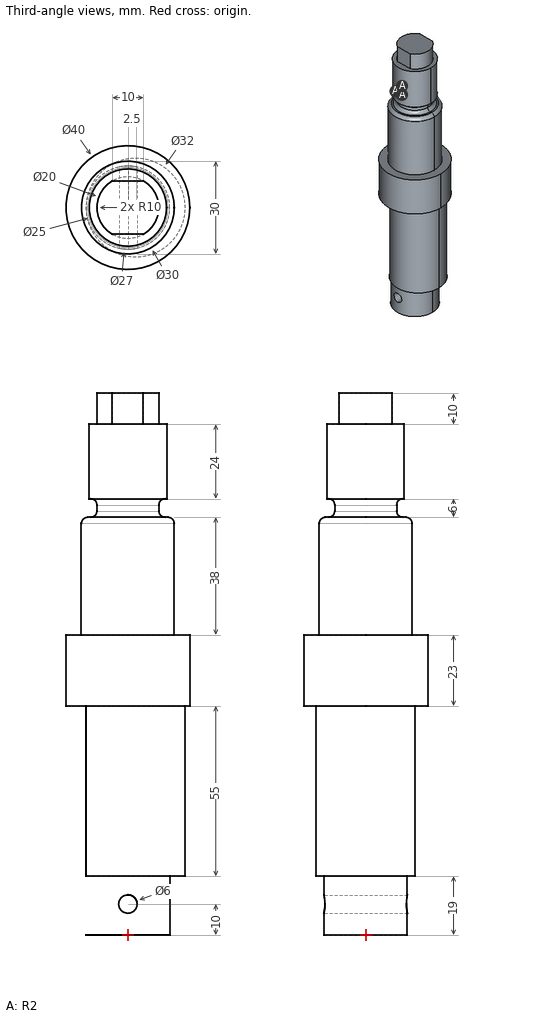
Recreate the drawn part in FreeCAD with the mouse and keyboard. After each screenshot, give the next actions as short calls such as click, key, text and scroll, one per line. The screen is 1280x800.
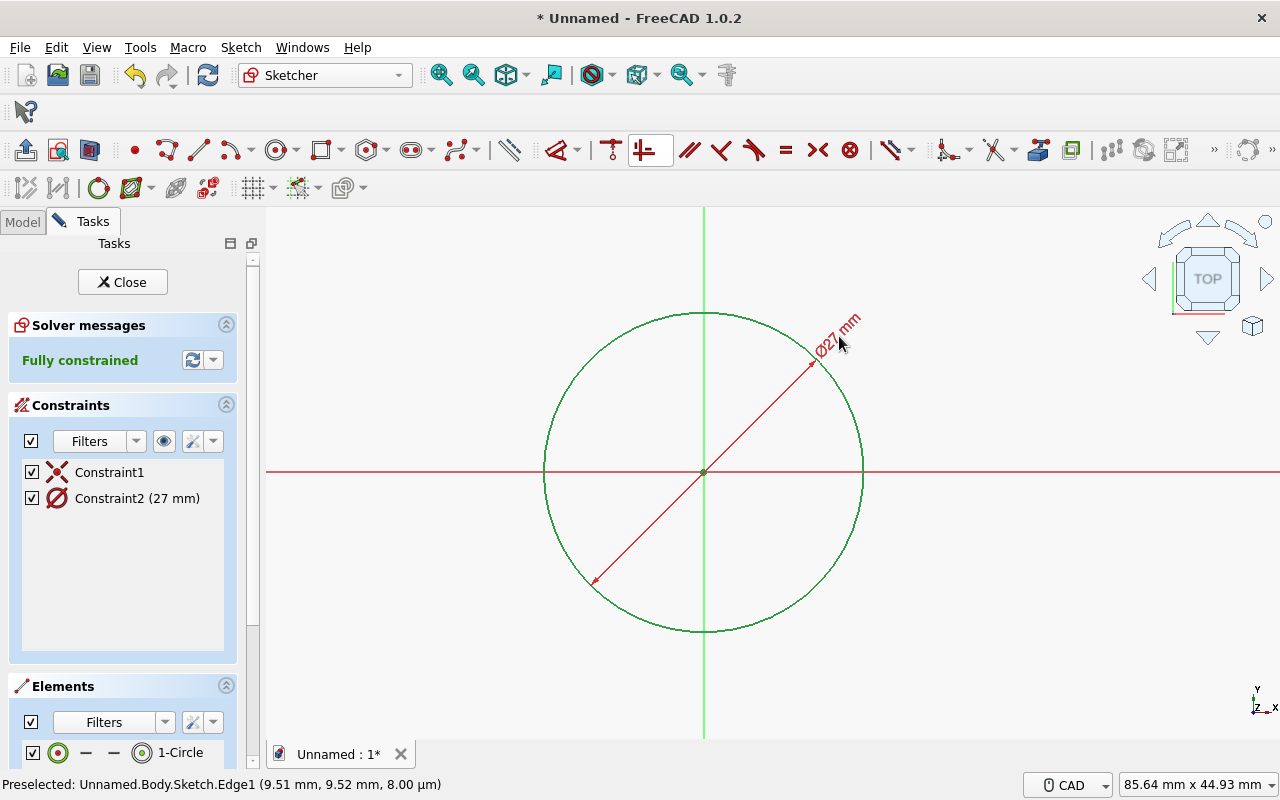
click(123, 282)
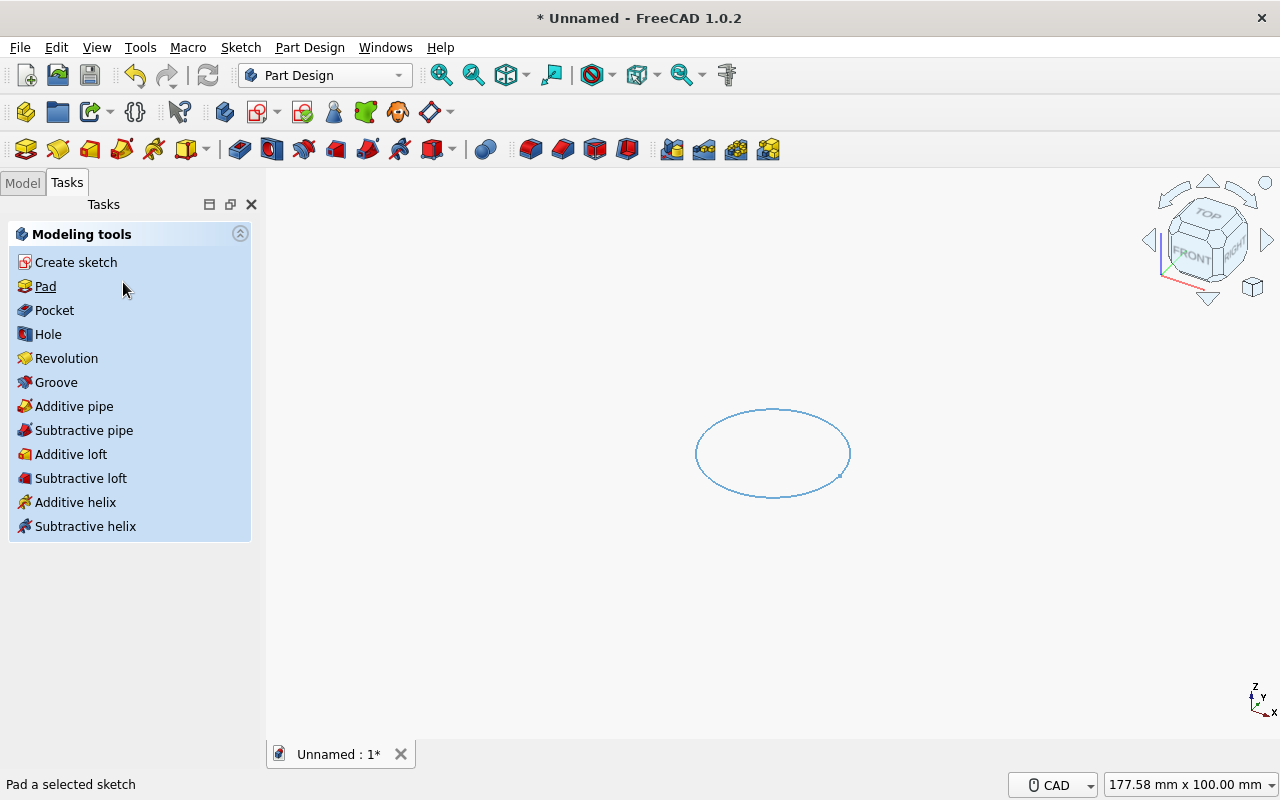
click(26, 150)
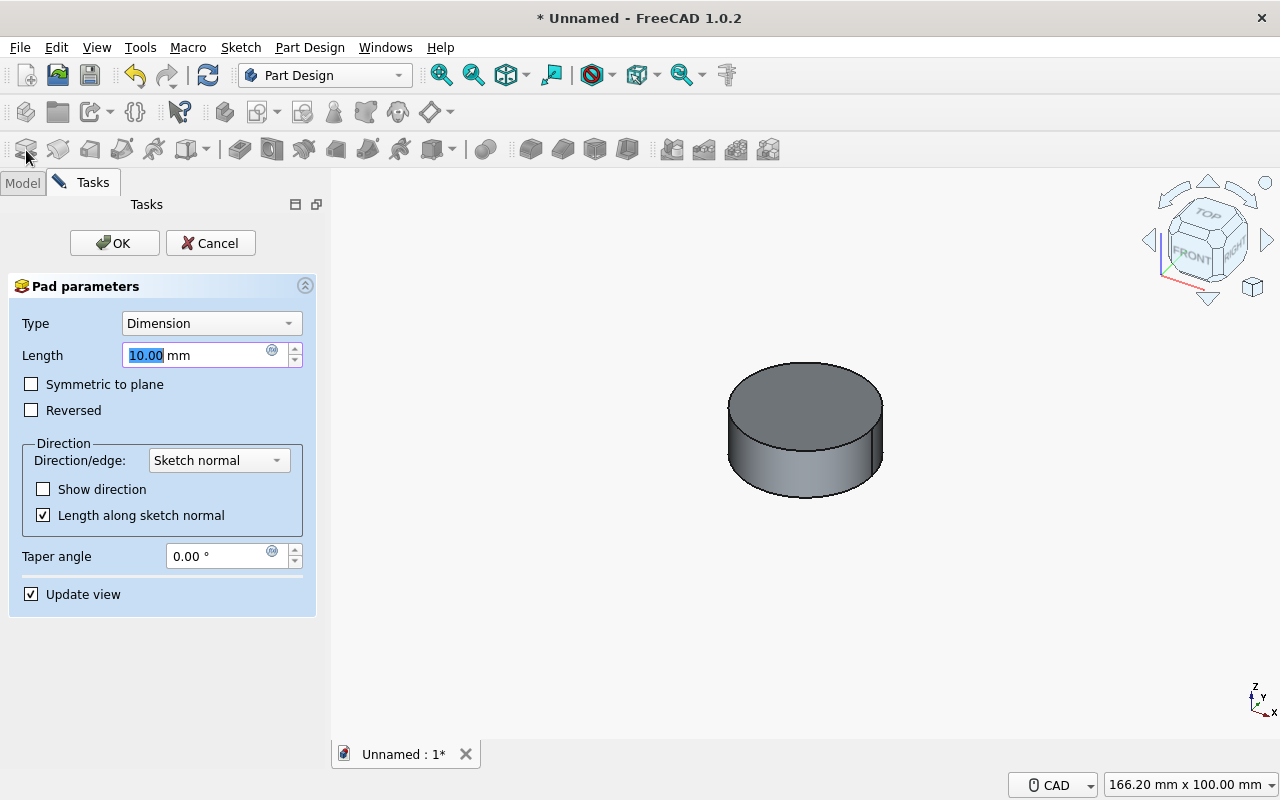
text(19)
key(Tab)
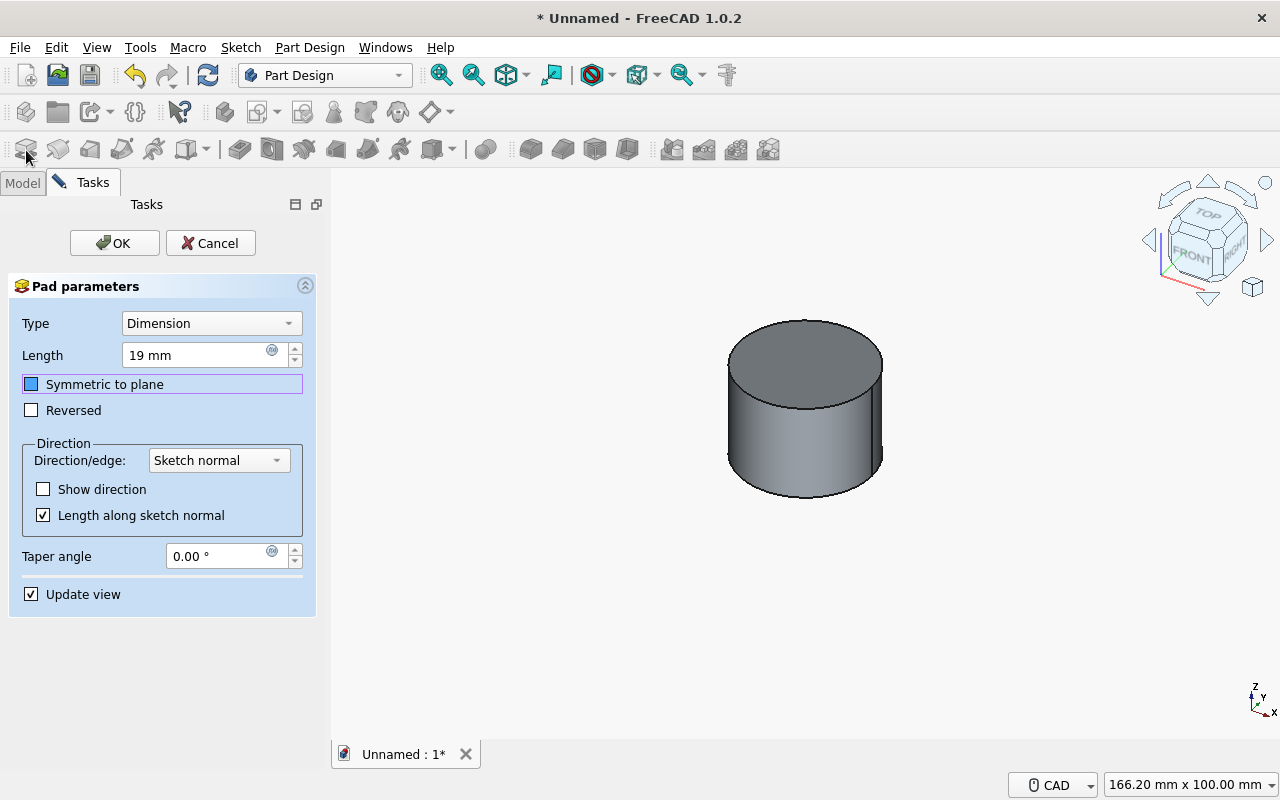
click(115, 243)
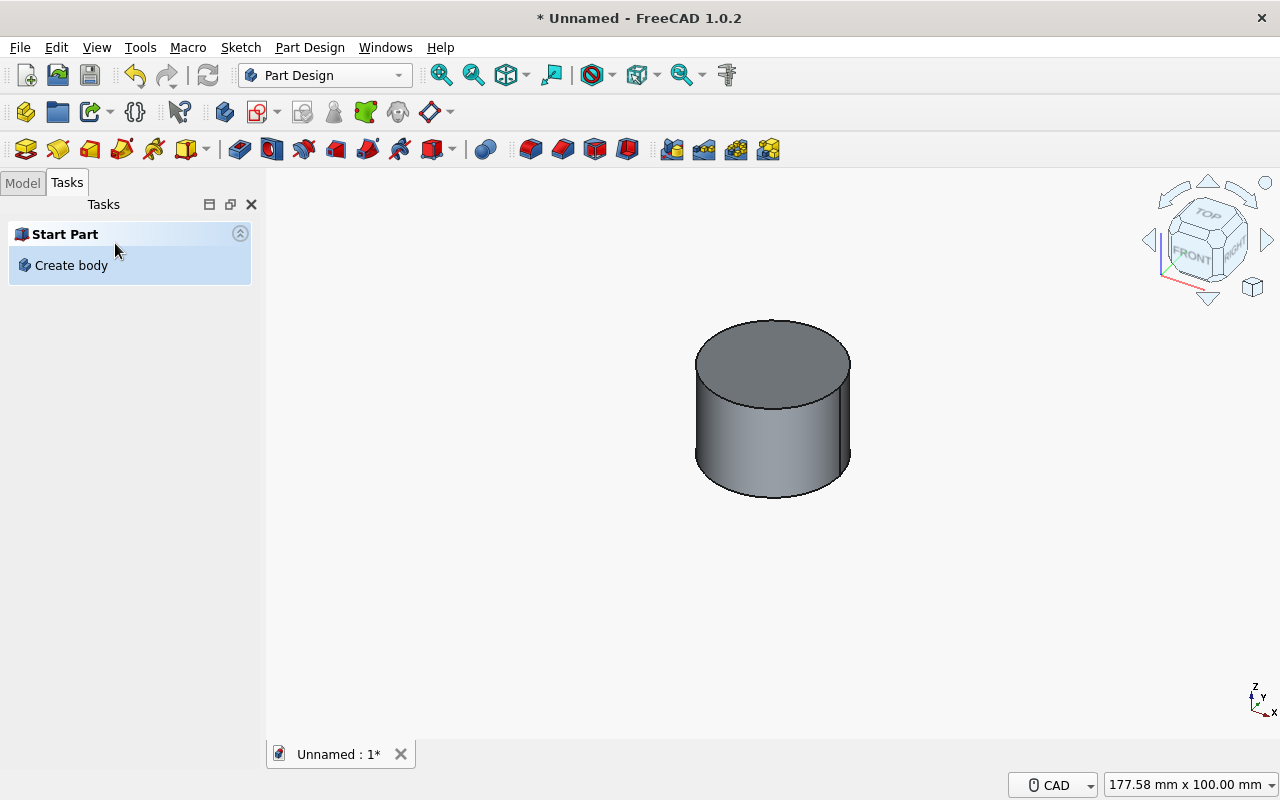
click(442, 76)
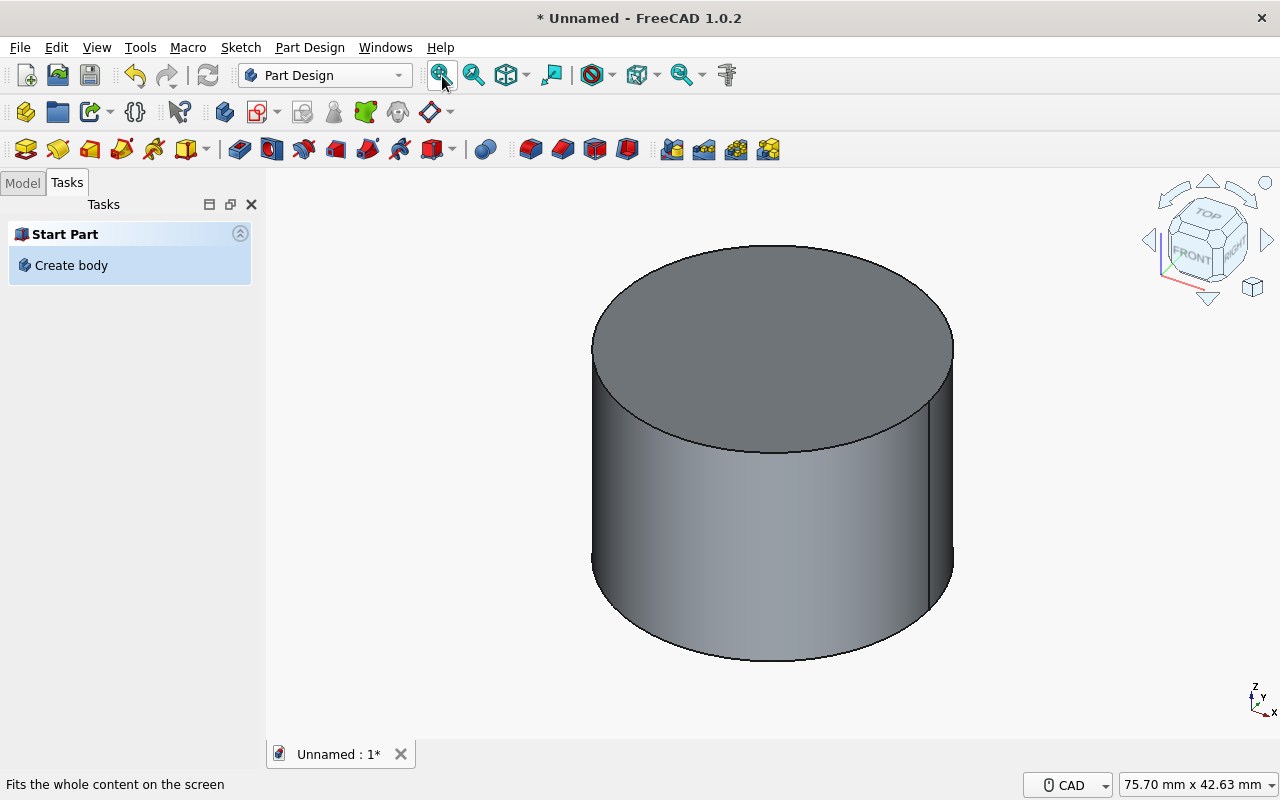
click(773, 348)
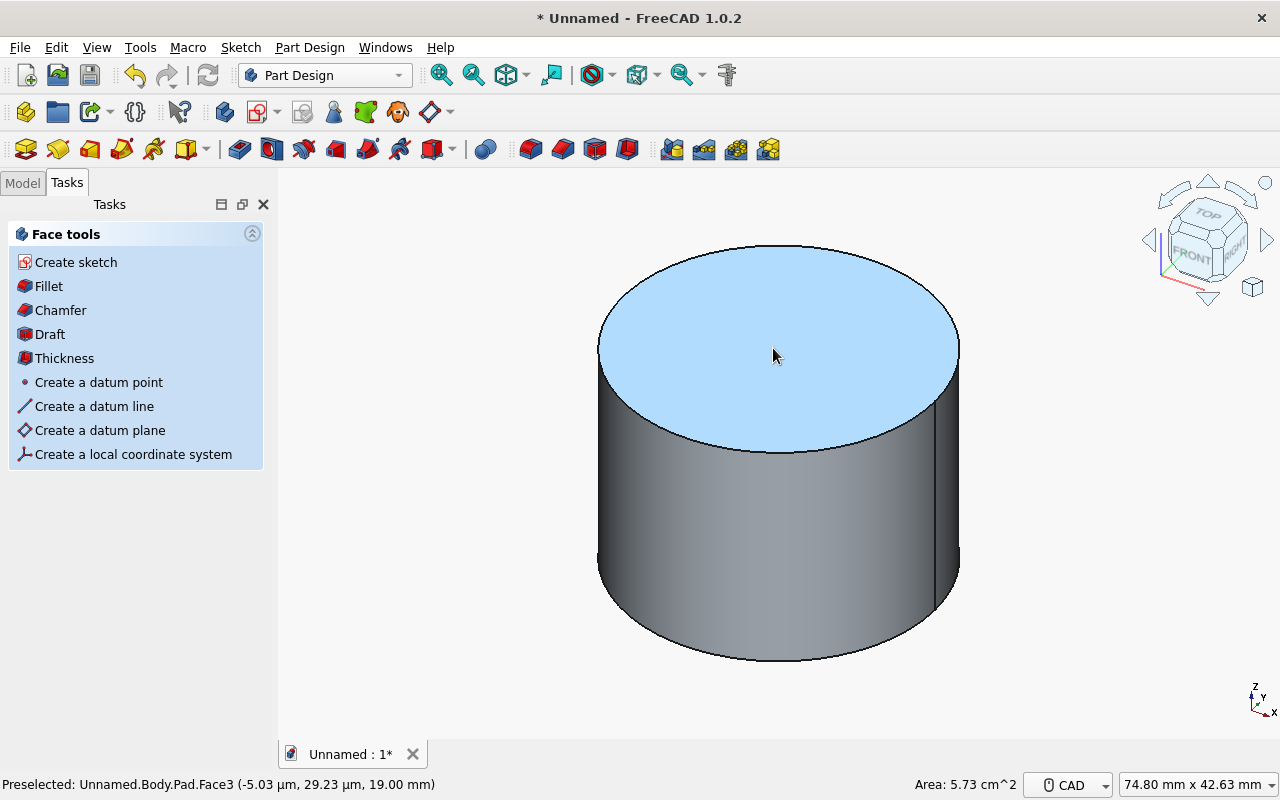
click(258, 112)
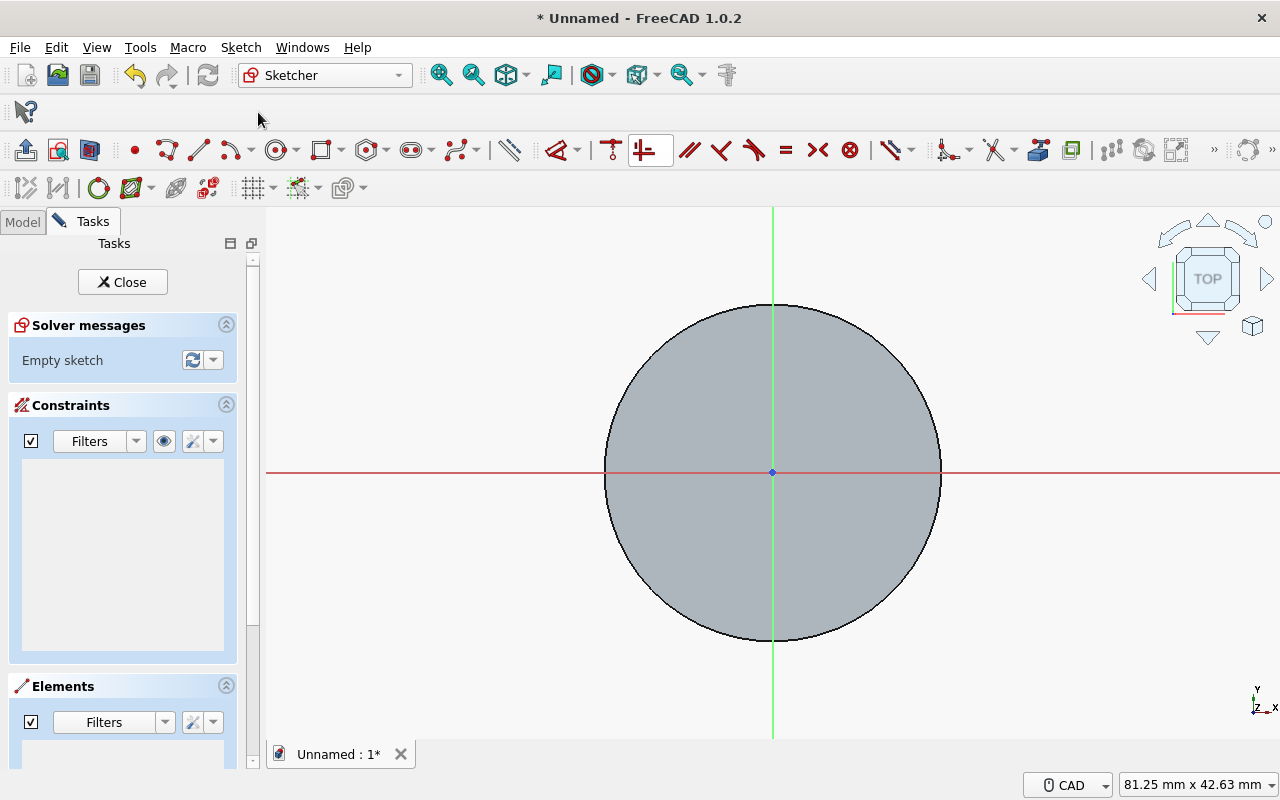
key(g)
key(c)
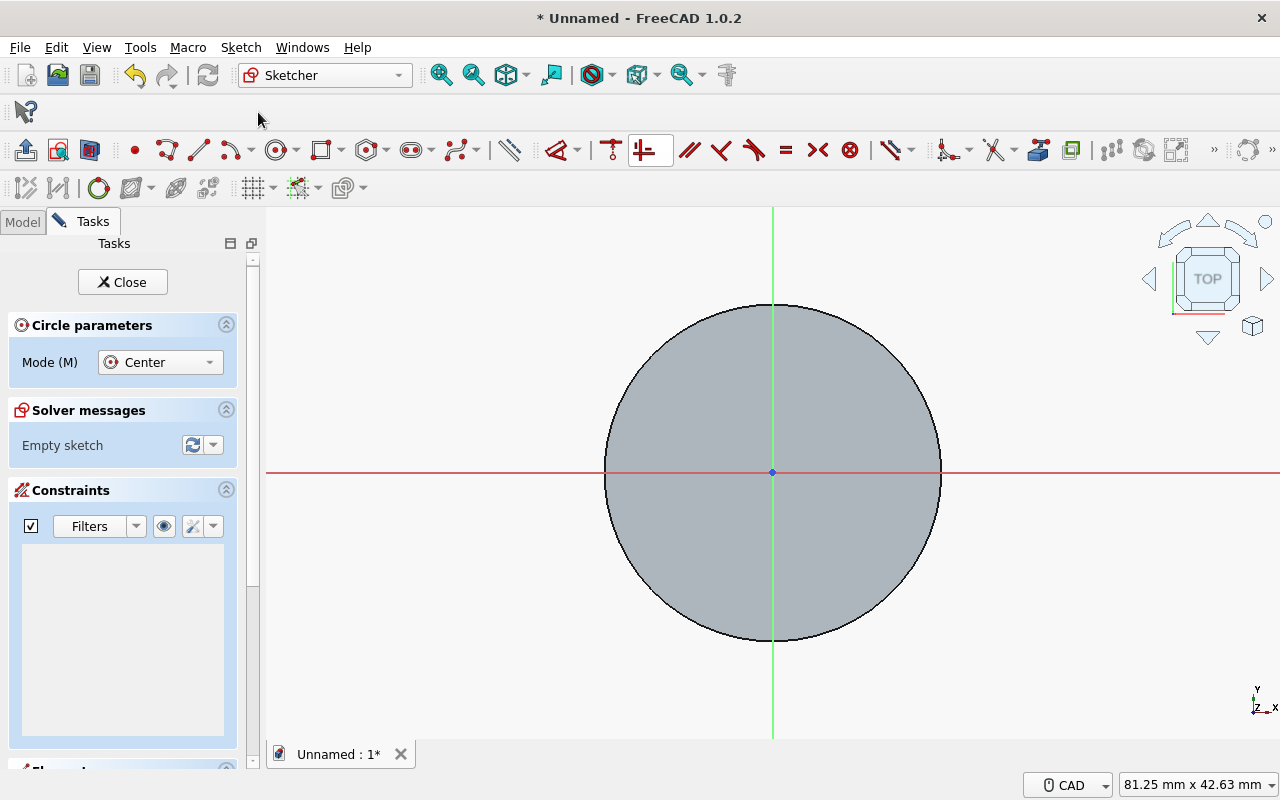
click(804, 473)
click(945, 332)
key(Escape)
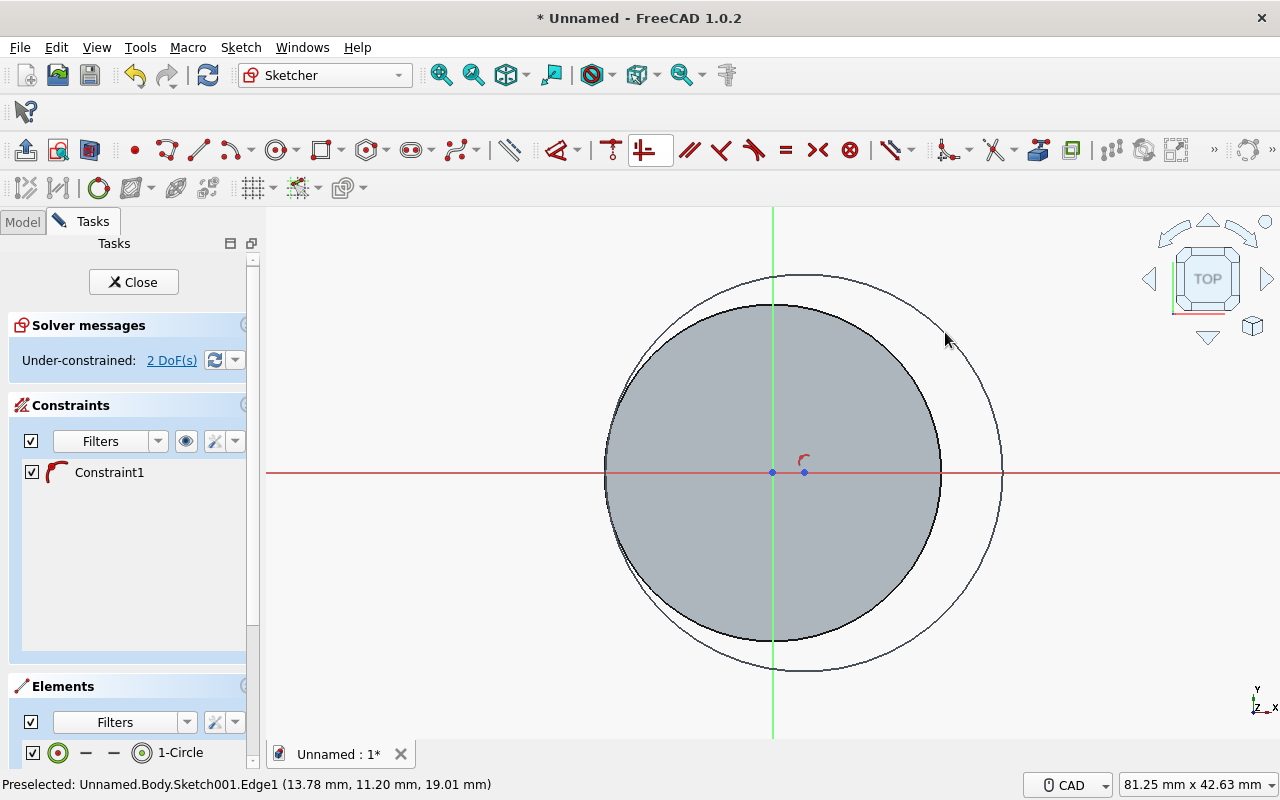
key(d)